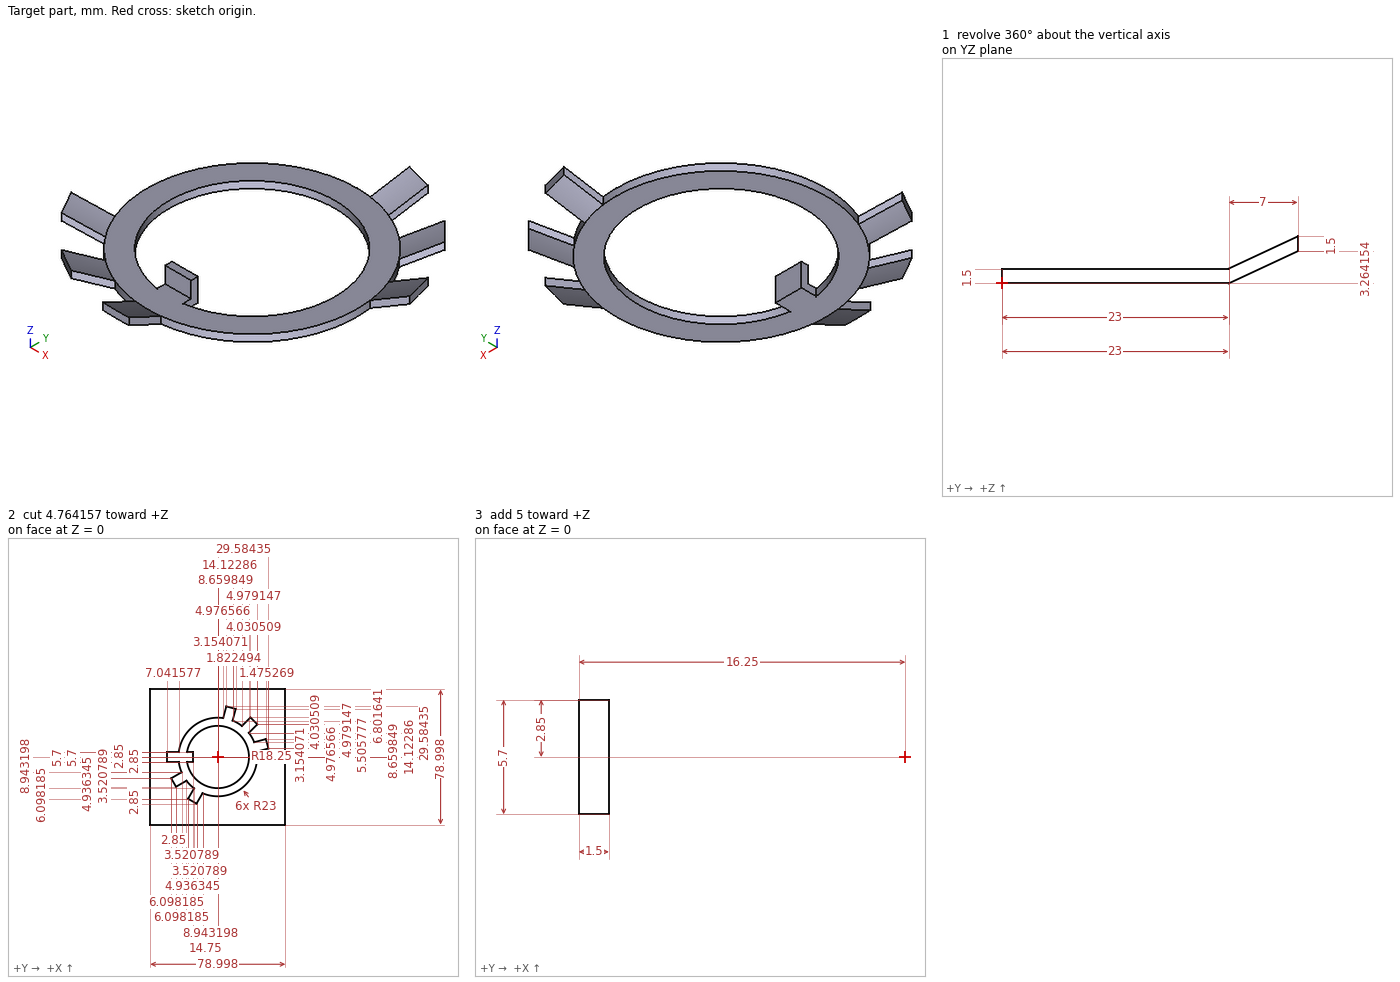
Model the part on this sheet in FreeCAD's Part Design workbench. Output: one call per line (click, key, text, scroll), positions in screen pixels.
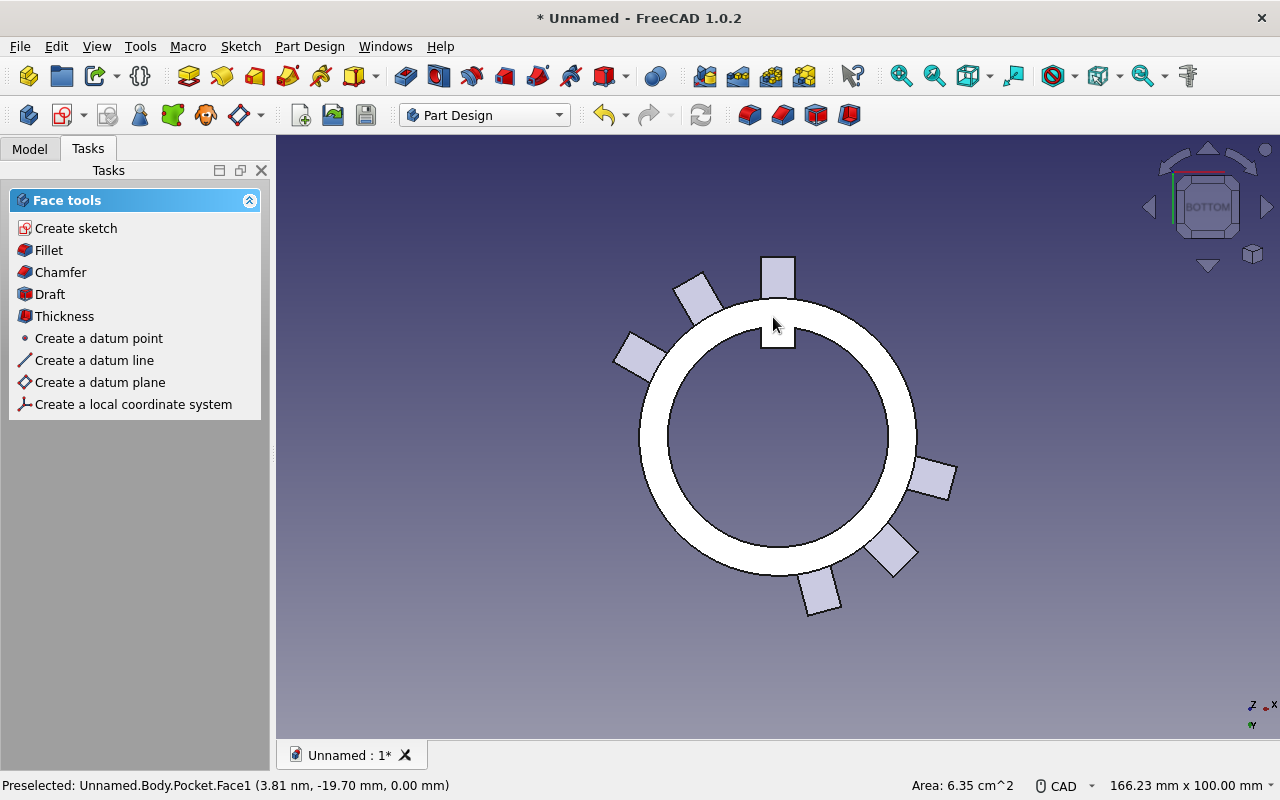
click(62, 116)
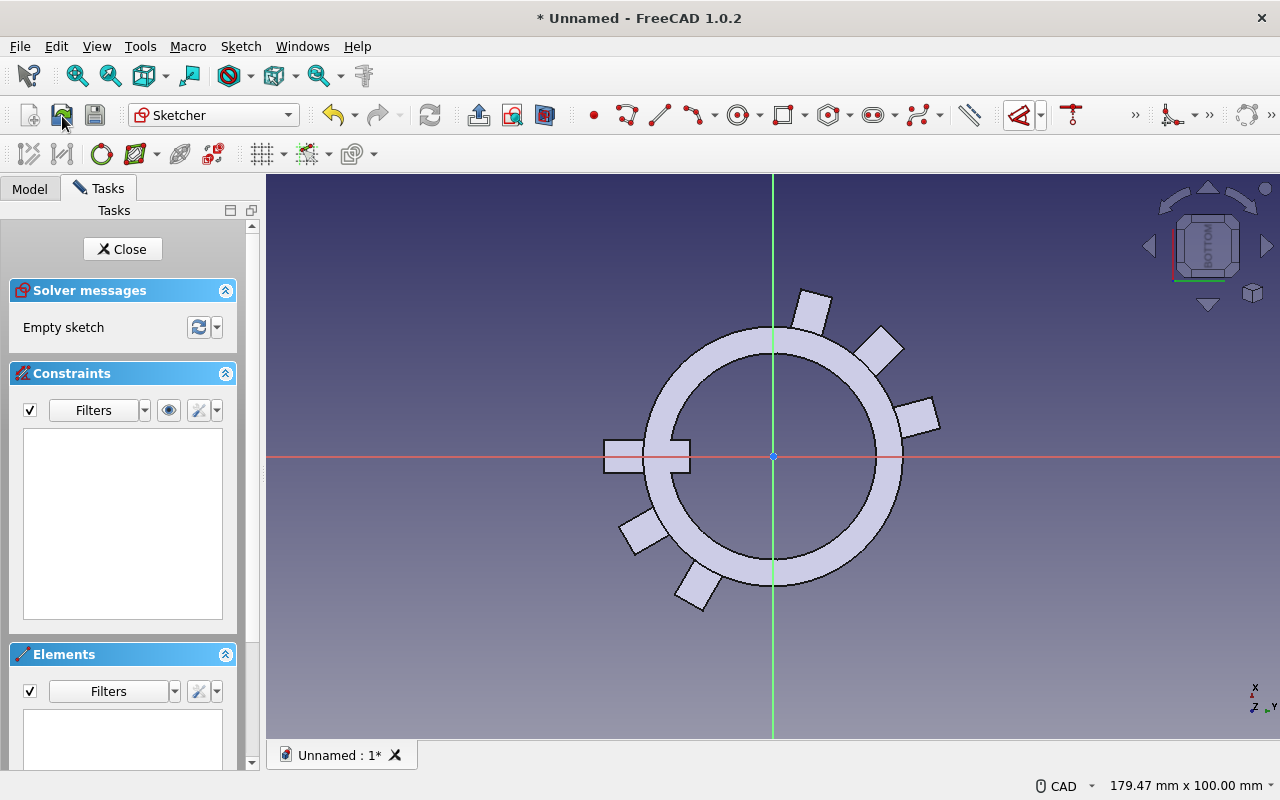
scroll(684, 457, up, 12)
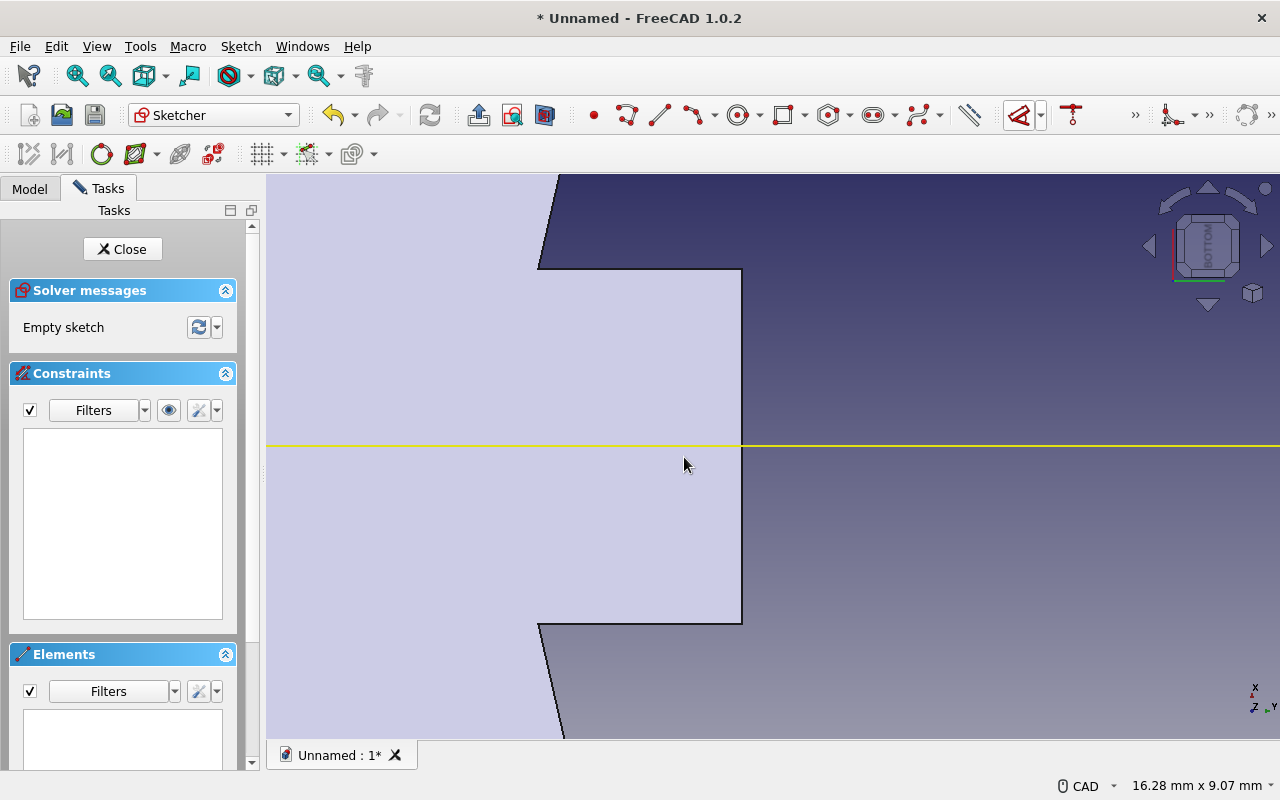
click(782, 116)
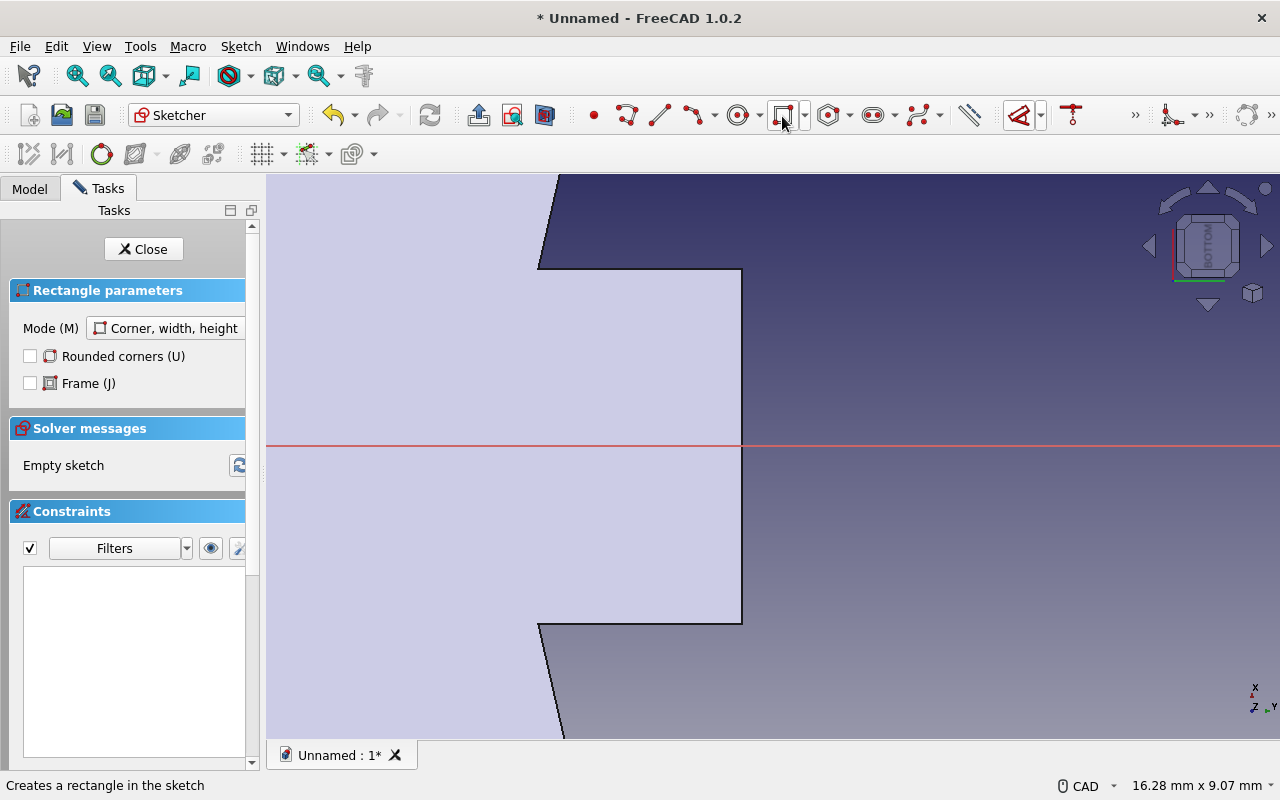
click(649, 269)
move(742, 624)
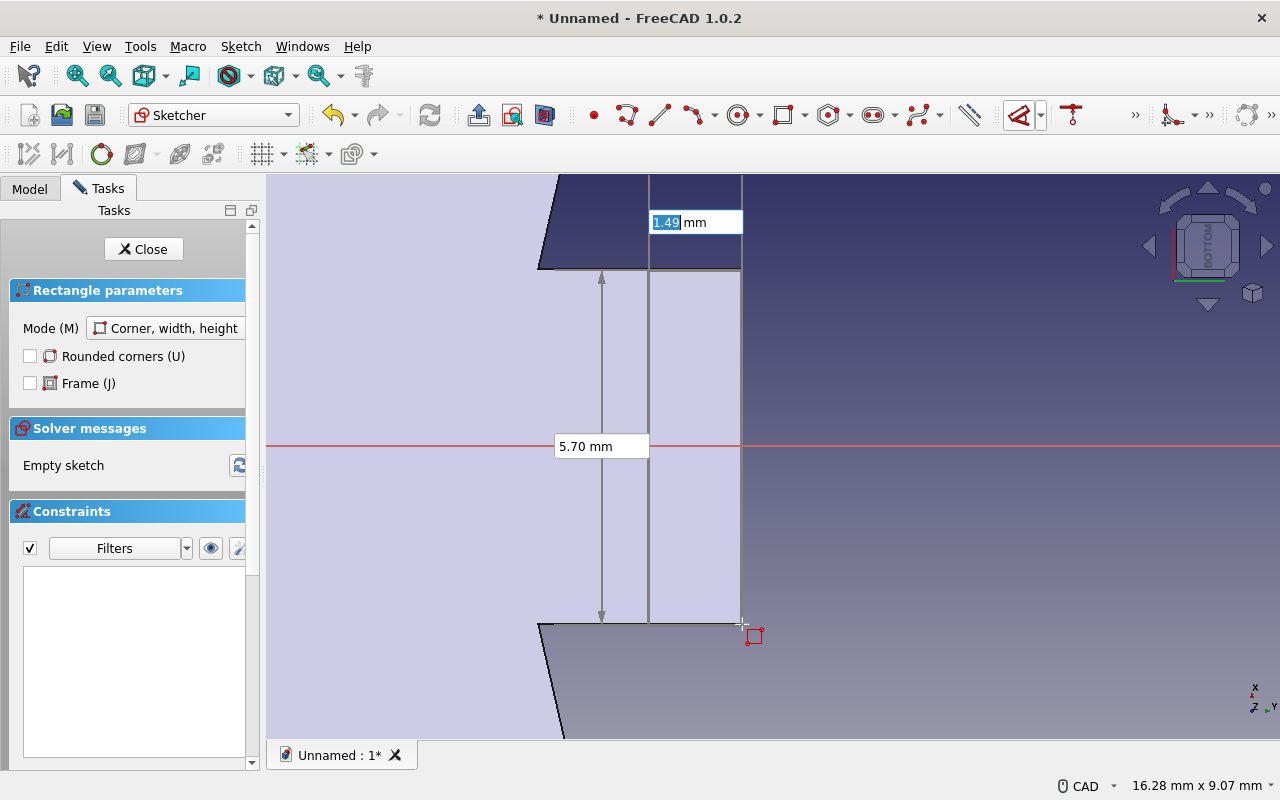
text(1.5)
key(Tab)
text(5.7)
key(Return)
key(Escape)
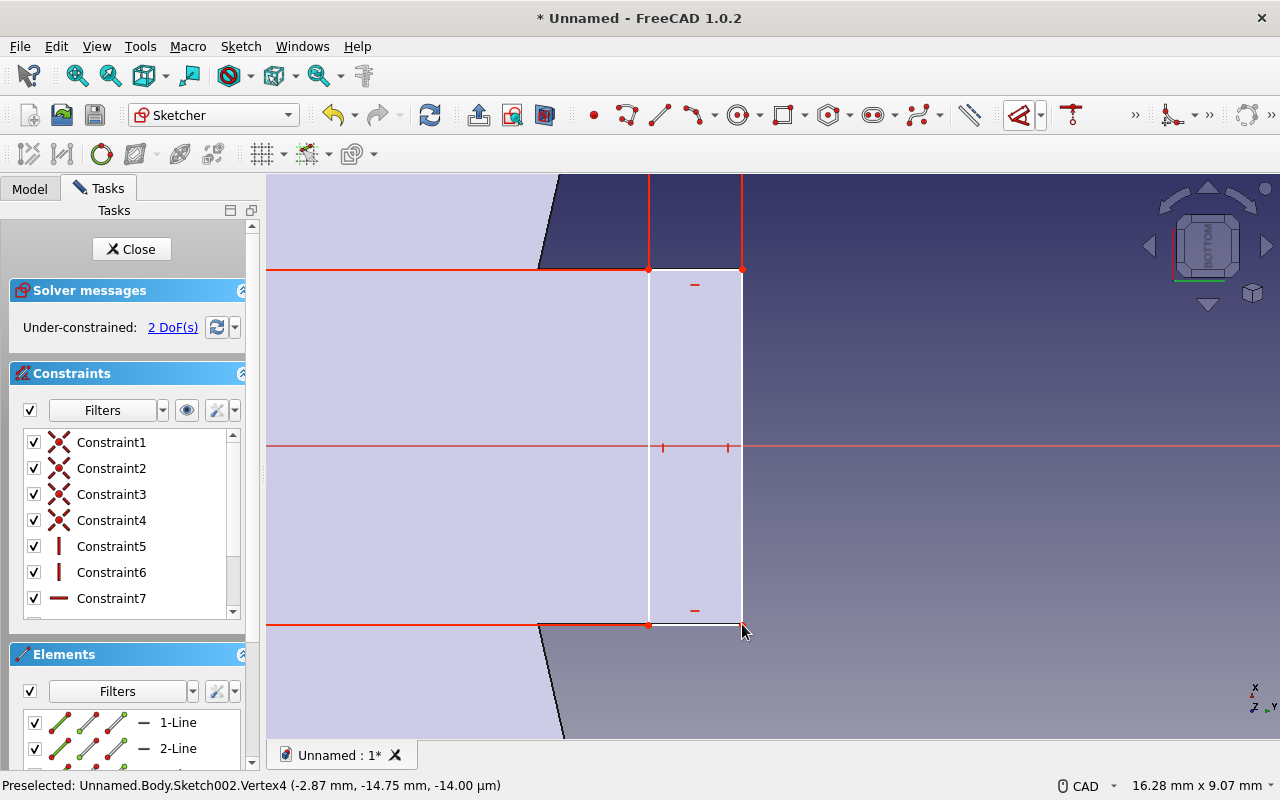
click(649, 270)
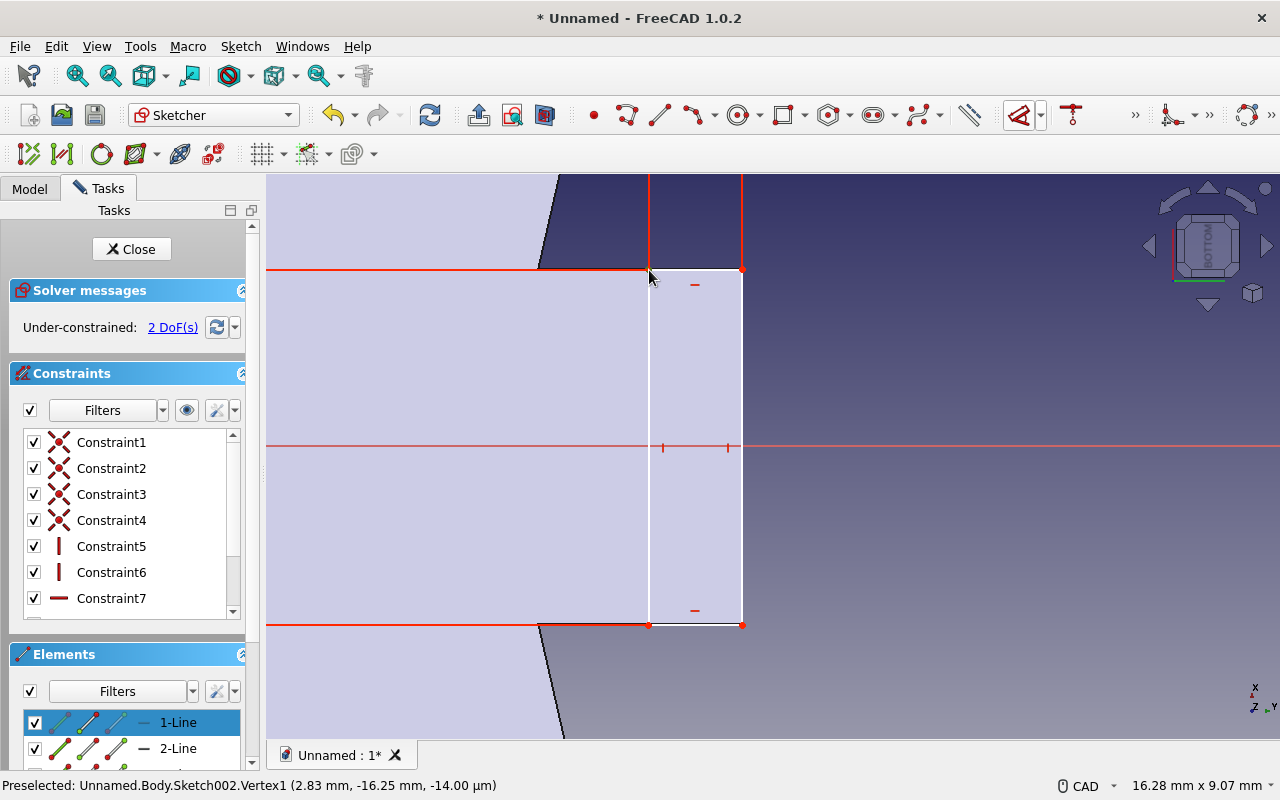
key(i)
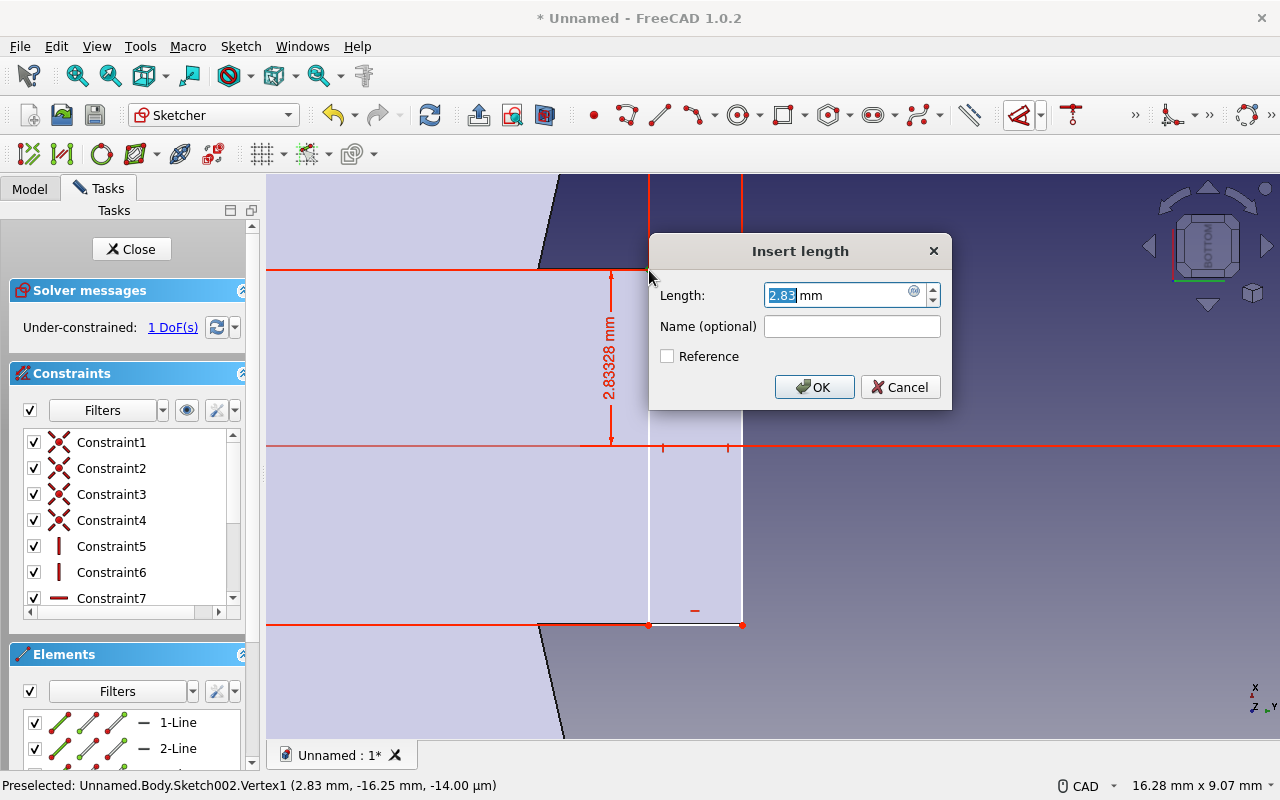
text(2.85)
key(Return)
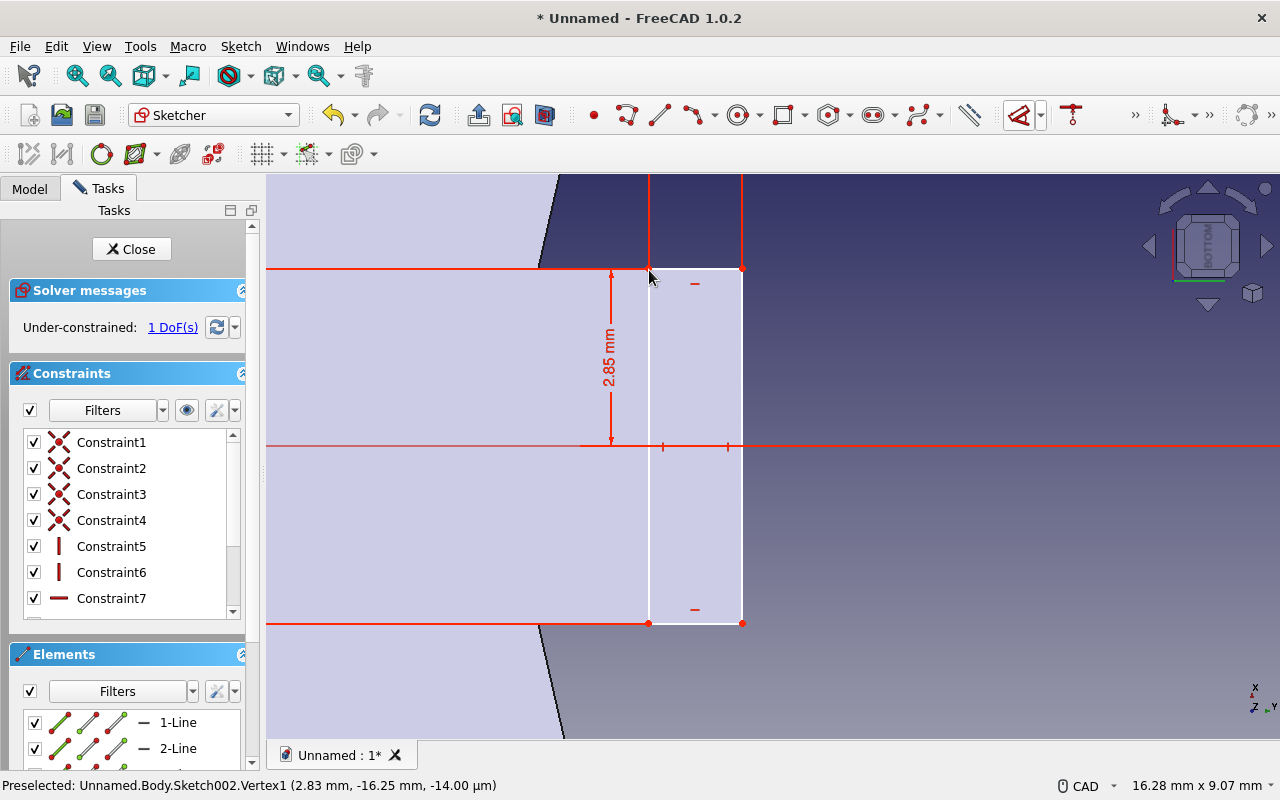
click(649, 269)